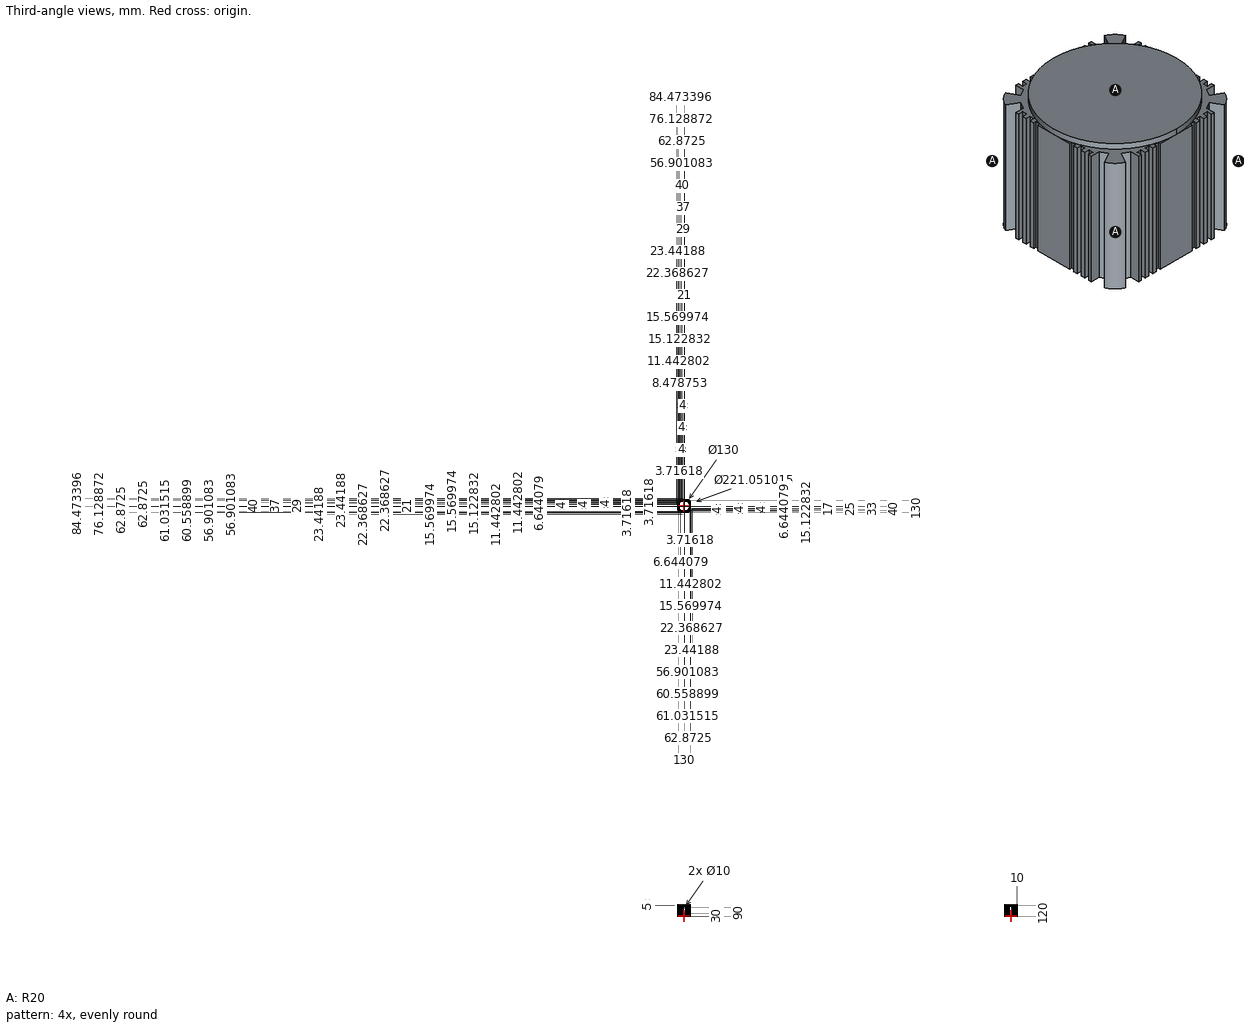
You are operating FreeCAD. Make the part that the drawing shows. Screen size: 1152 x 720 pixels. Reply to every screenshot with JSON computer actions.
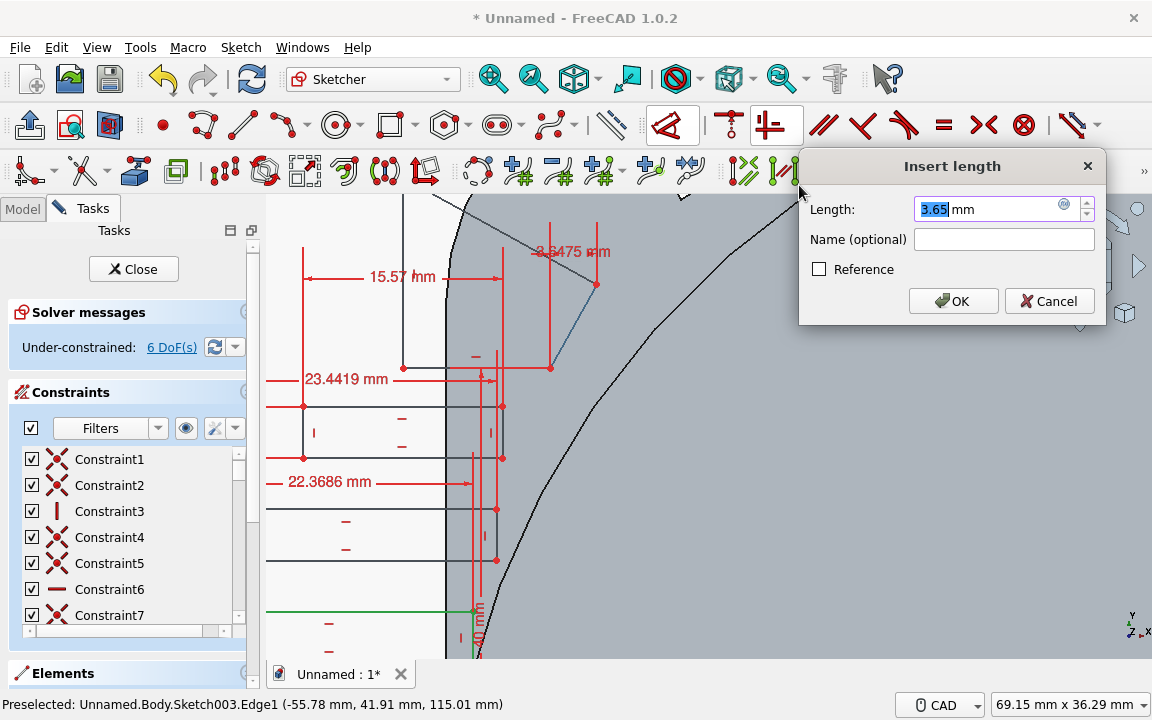
{"action": "type", "text": "3.71618"}
{"action": "key", "text": "Return"}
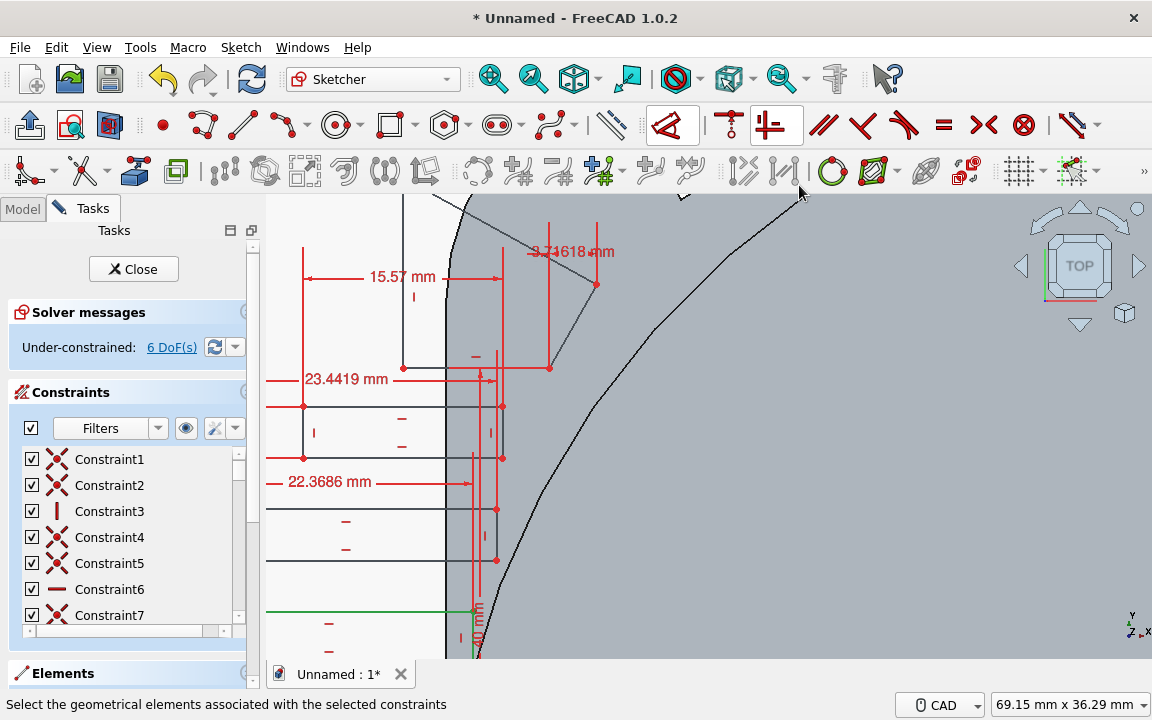
{"action": "left_click", "coordinate": [403, 235]}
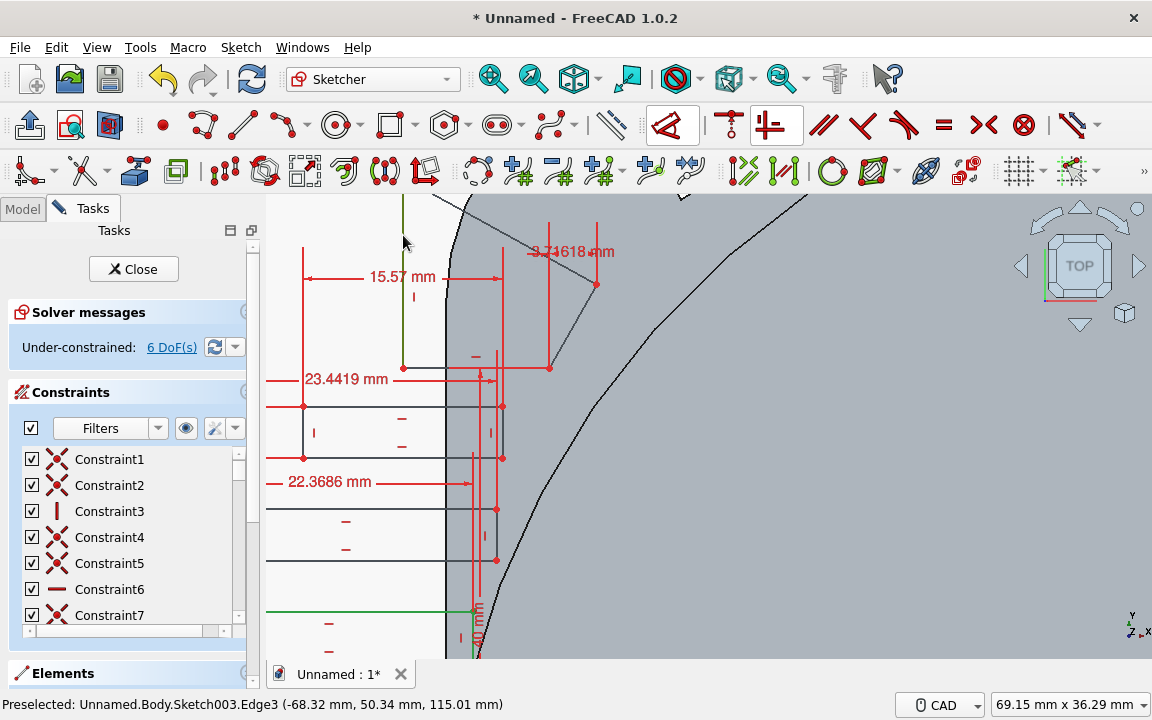
{"action": "left_click", "coordinate": [694, 126]}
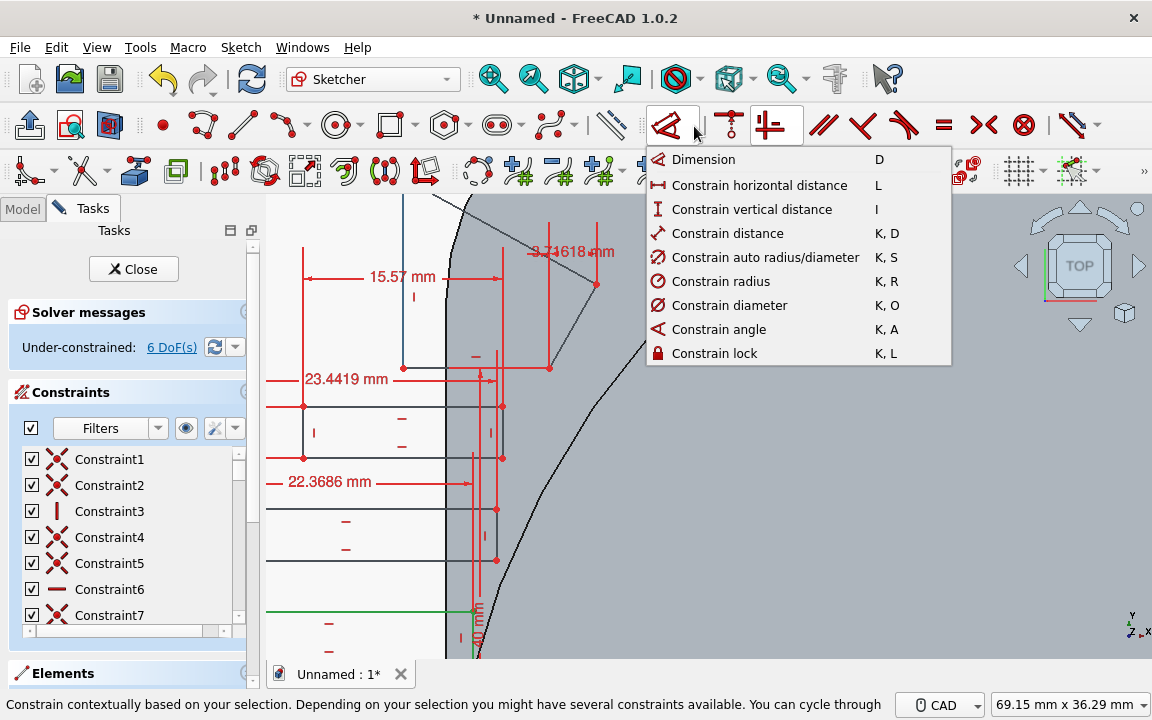
{"action": "left_click", "coordinate": [799, 209]}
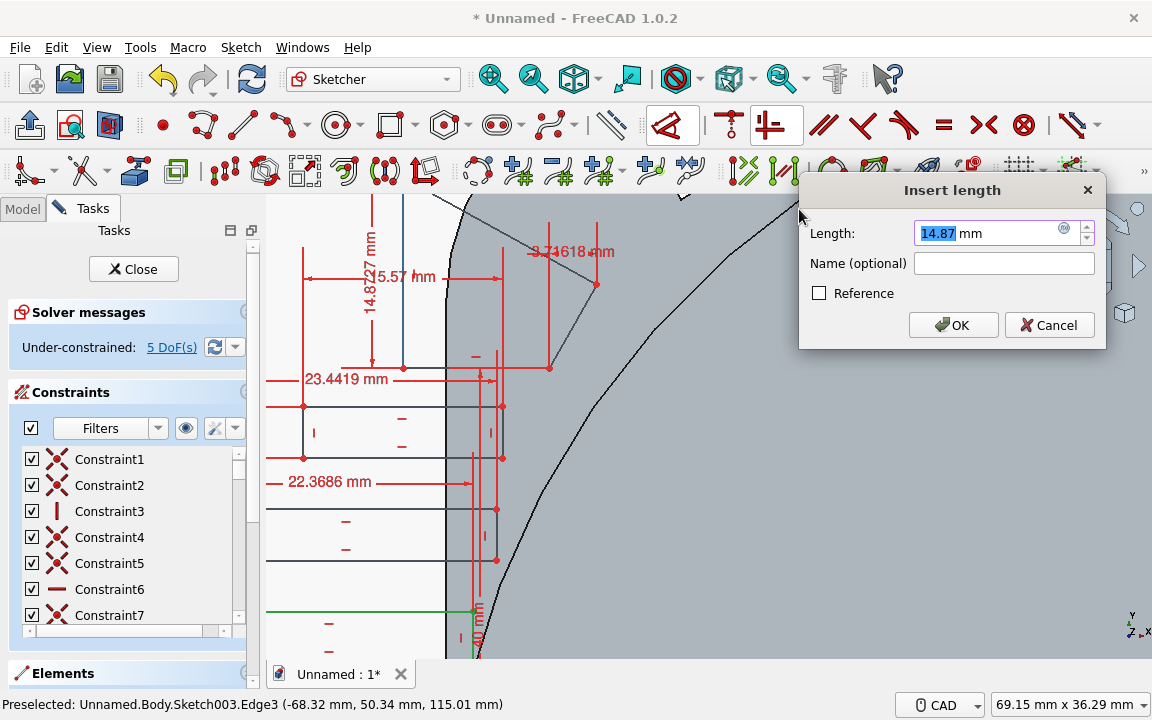
{"action": "type", "text": "15.122832"}
{"action": "key", "text": "Return"}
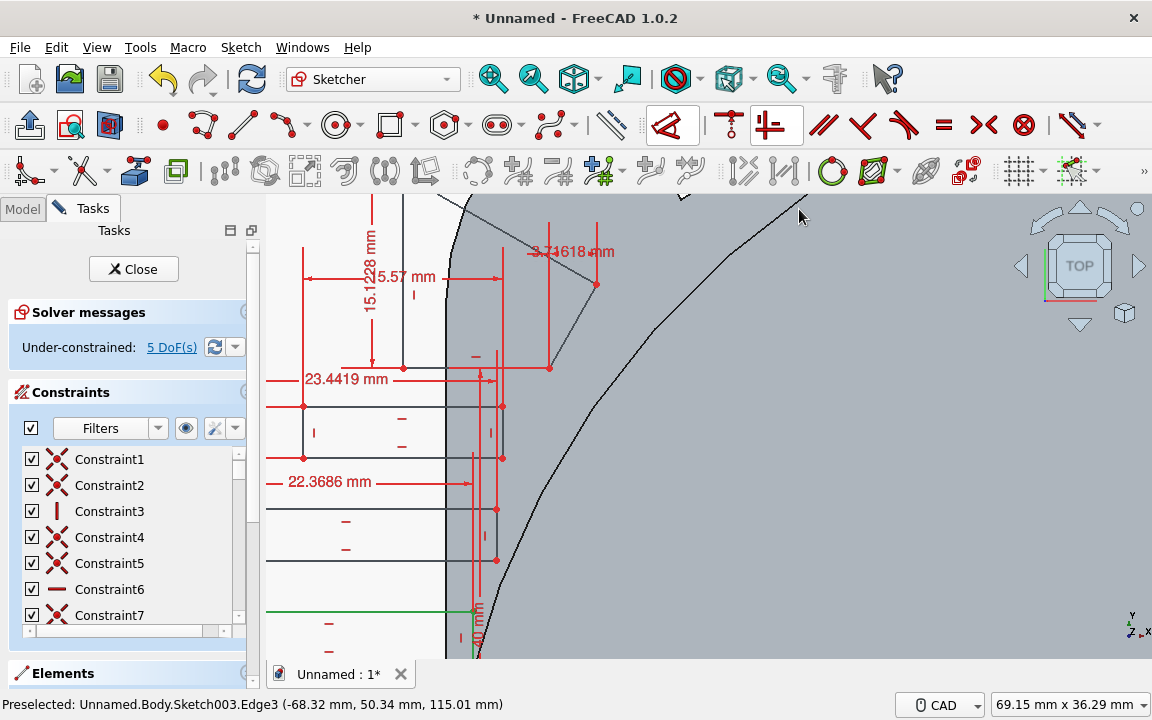
{"action": "left_click", "coordinate": [447, 368]}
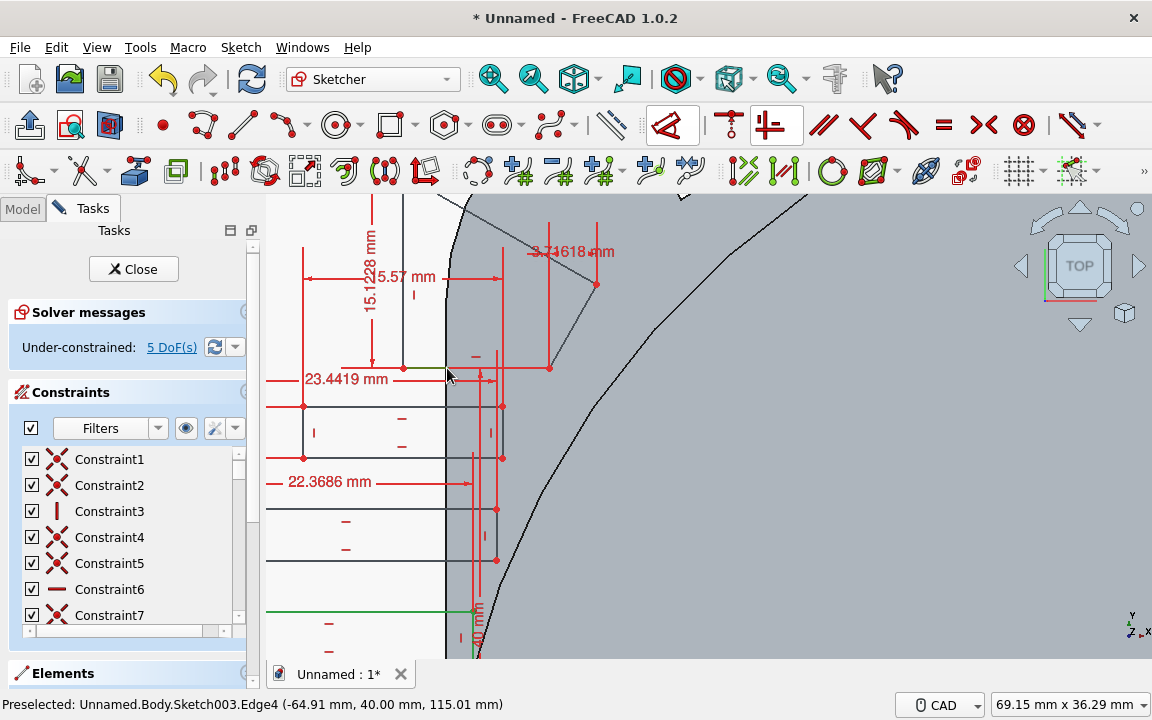
{"action": "left_click", "coordinate": [694, 126]}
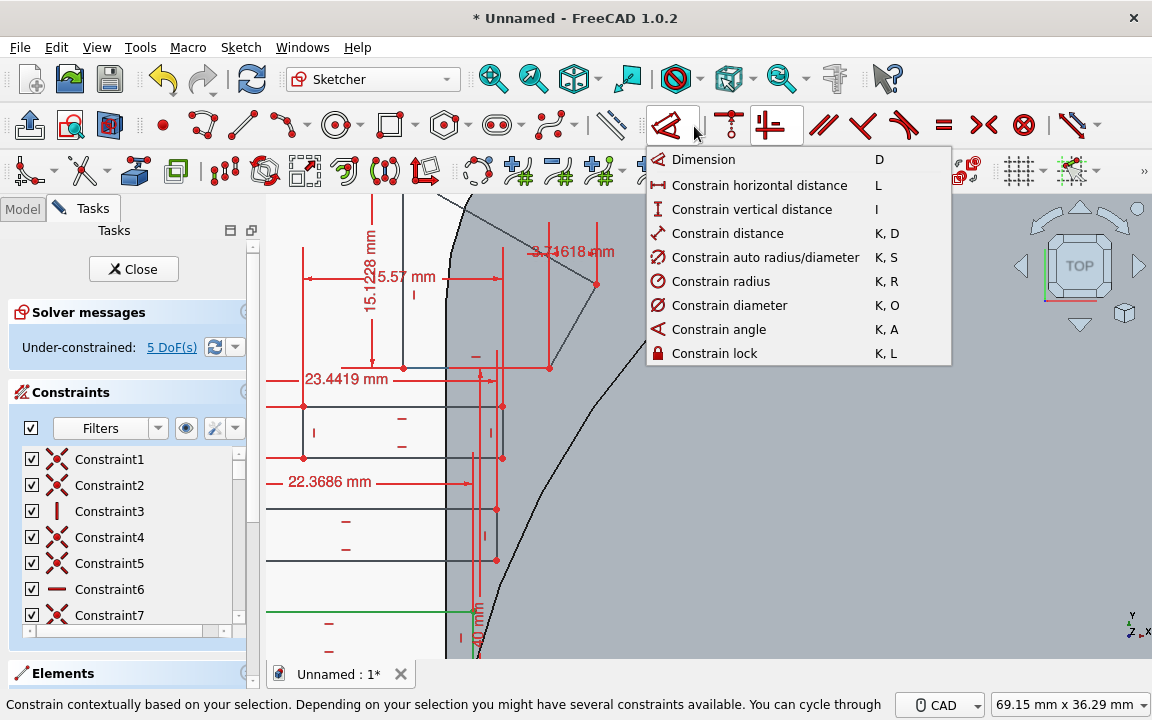
{"action": "left_click", "coordinate": [799, 185]}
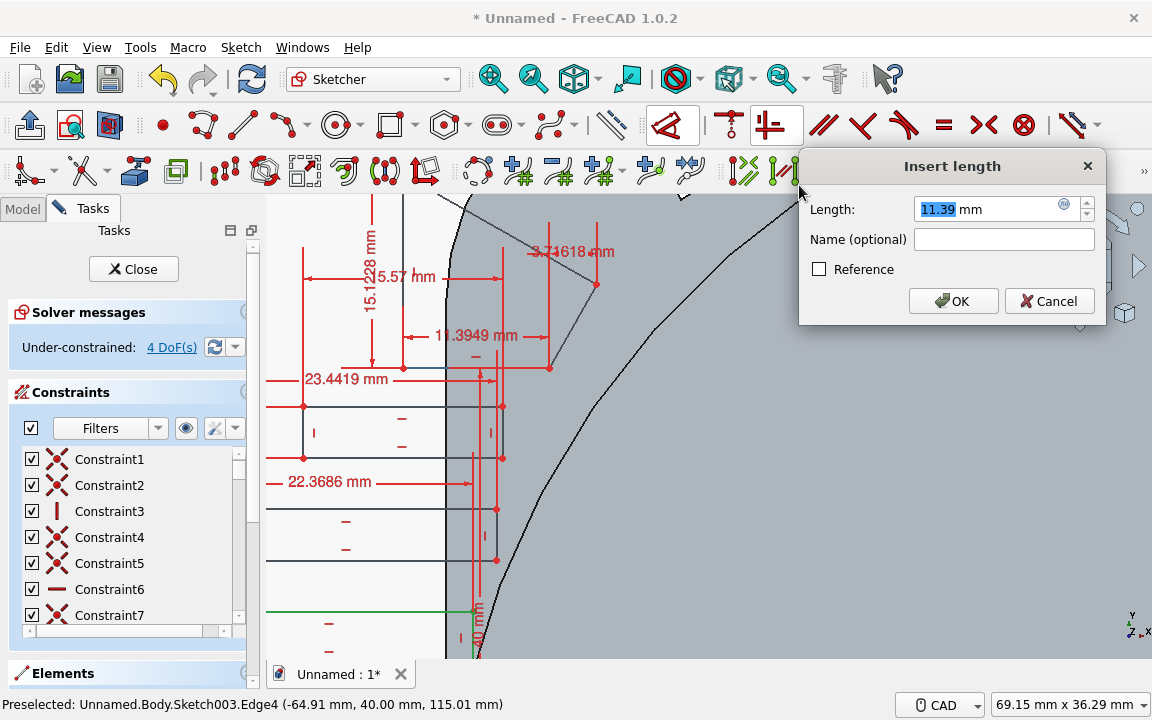
{"action": "type", "text": "11.442802"}
{"action": "key", "text": "Return"}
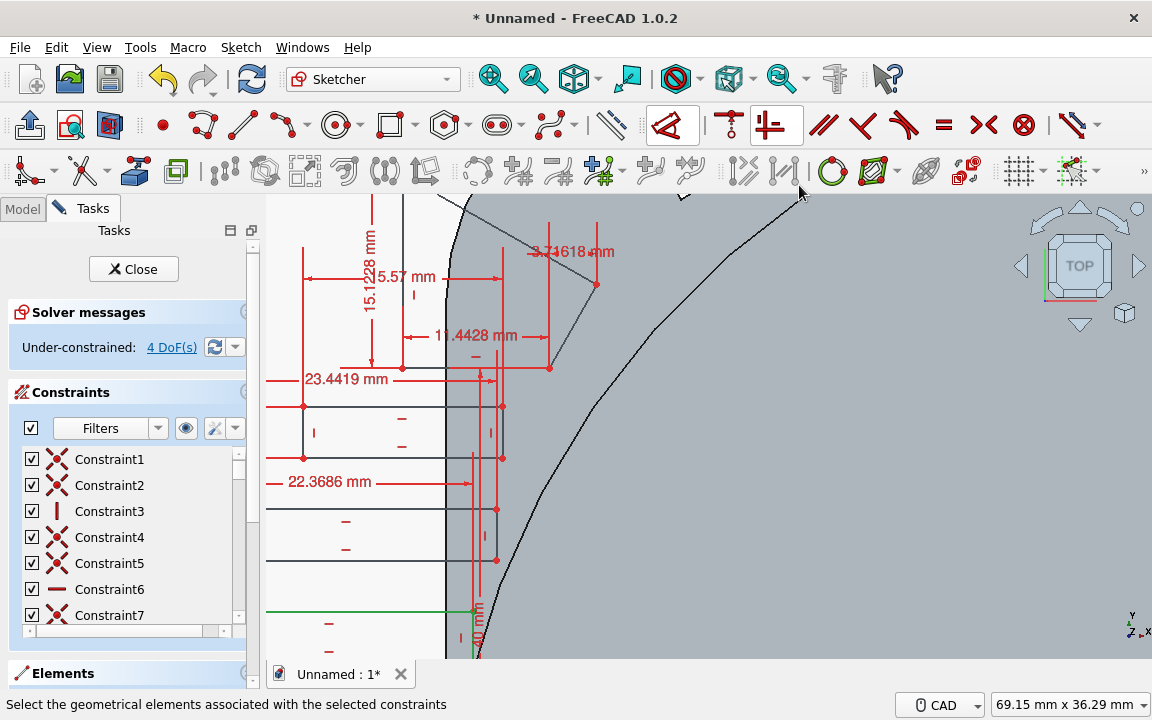
{"action": "left_click", "coordinate": [564, 343]}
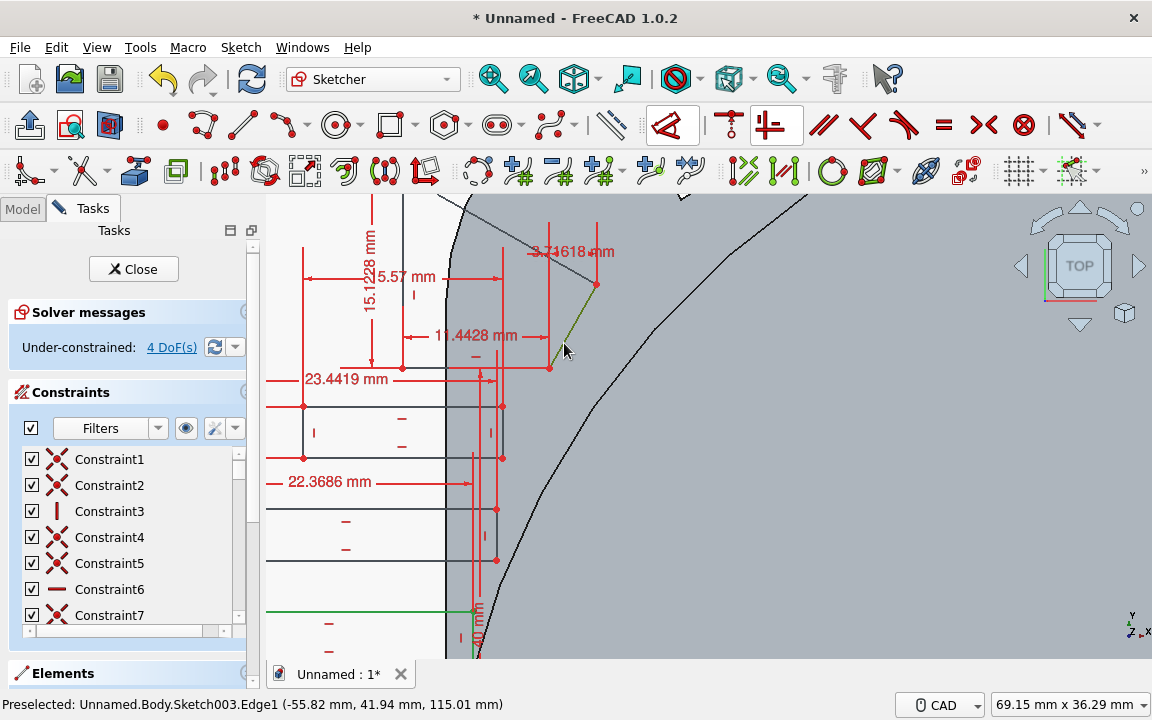
{"action": "left_click", "coordinate": [694, 126]}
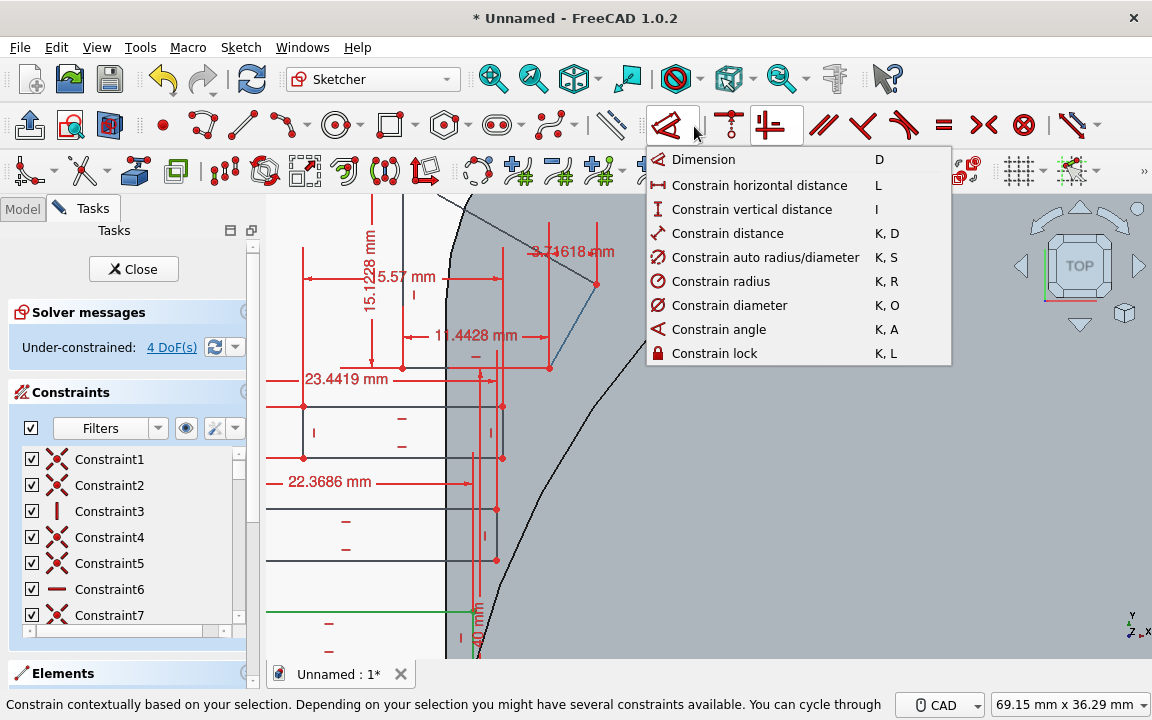
{"action": "left_click", "coordinate": [799, 209]}